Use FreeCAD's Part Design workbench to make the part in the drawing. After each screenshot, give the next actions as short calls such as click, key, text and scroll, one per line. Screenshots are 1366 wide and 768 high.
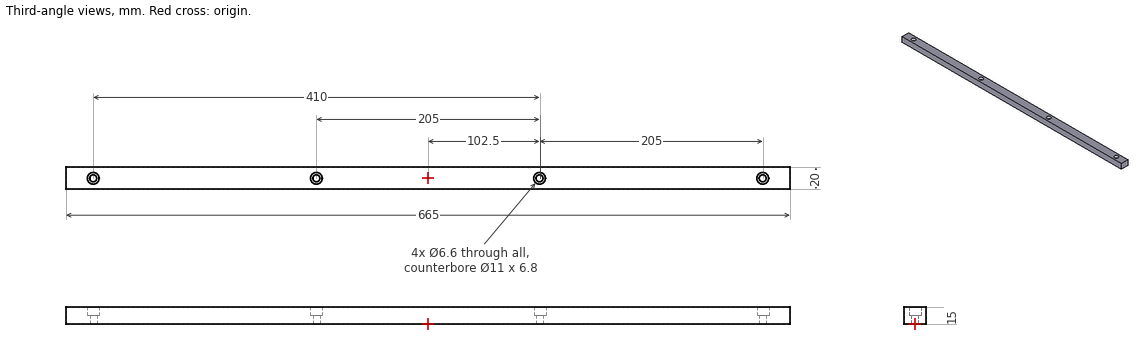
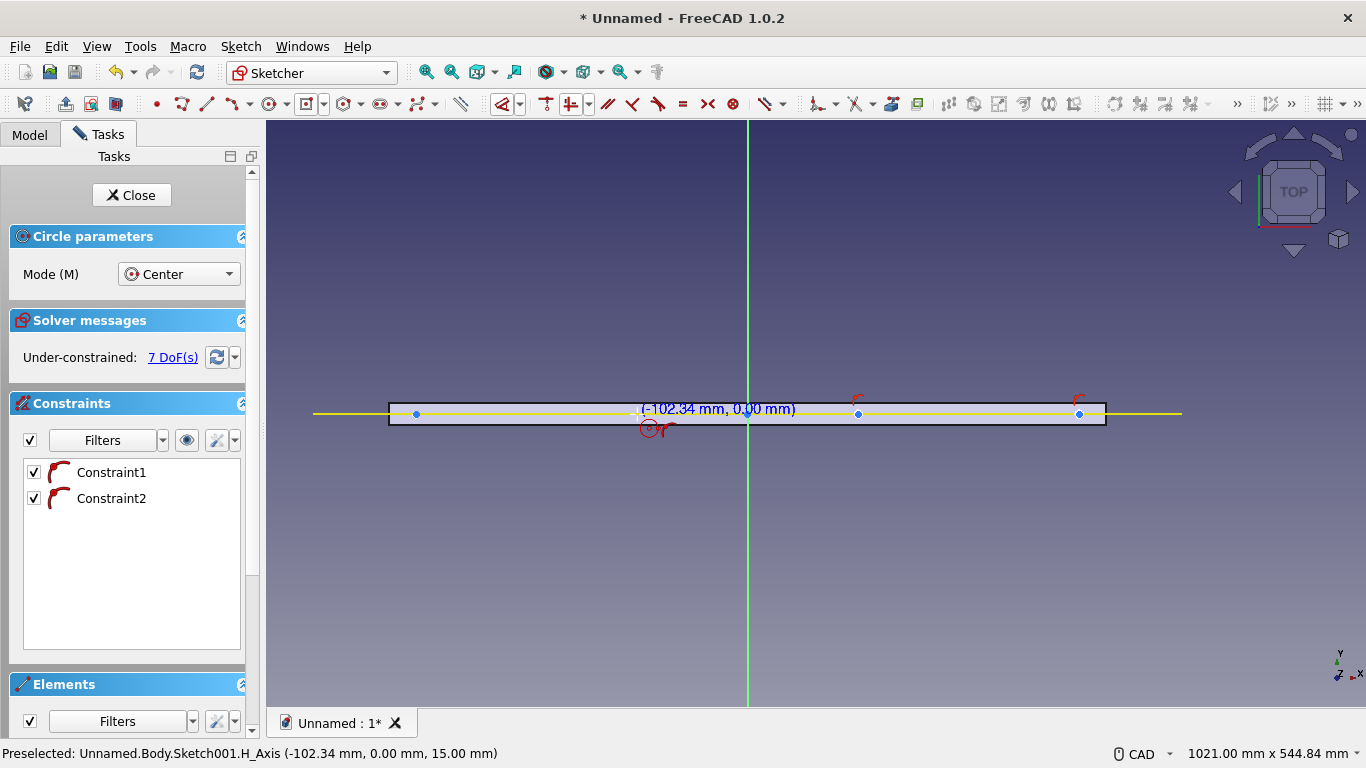
click(637, 414)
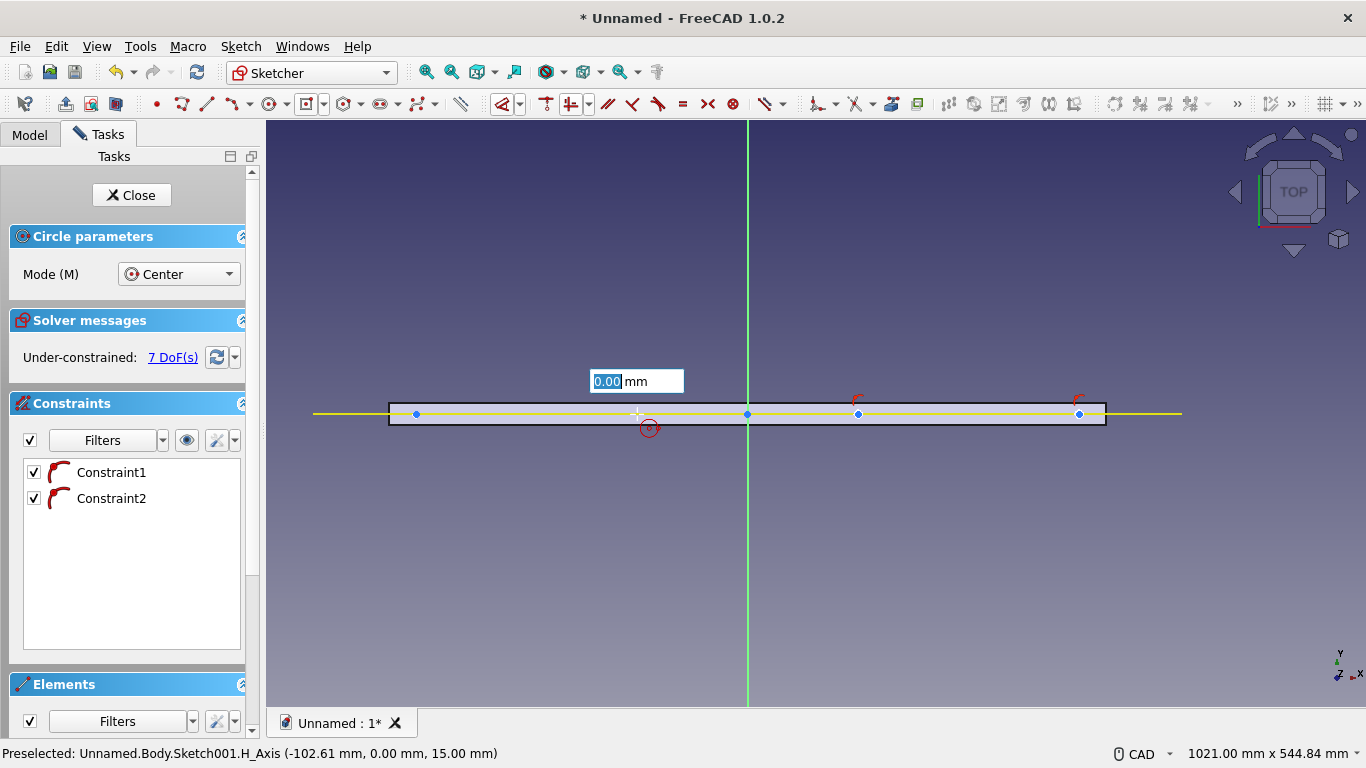
scroll(636, 417, up, 8)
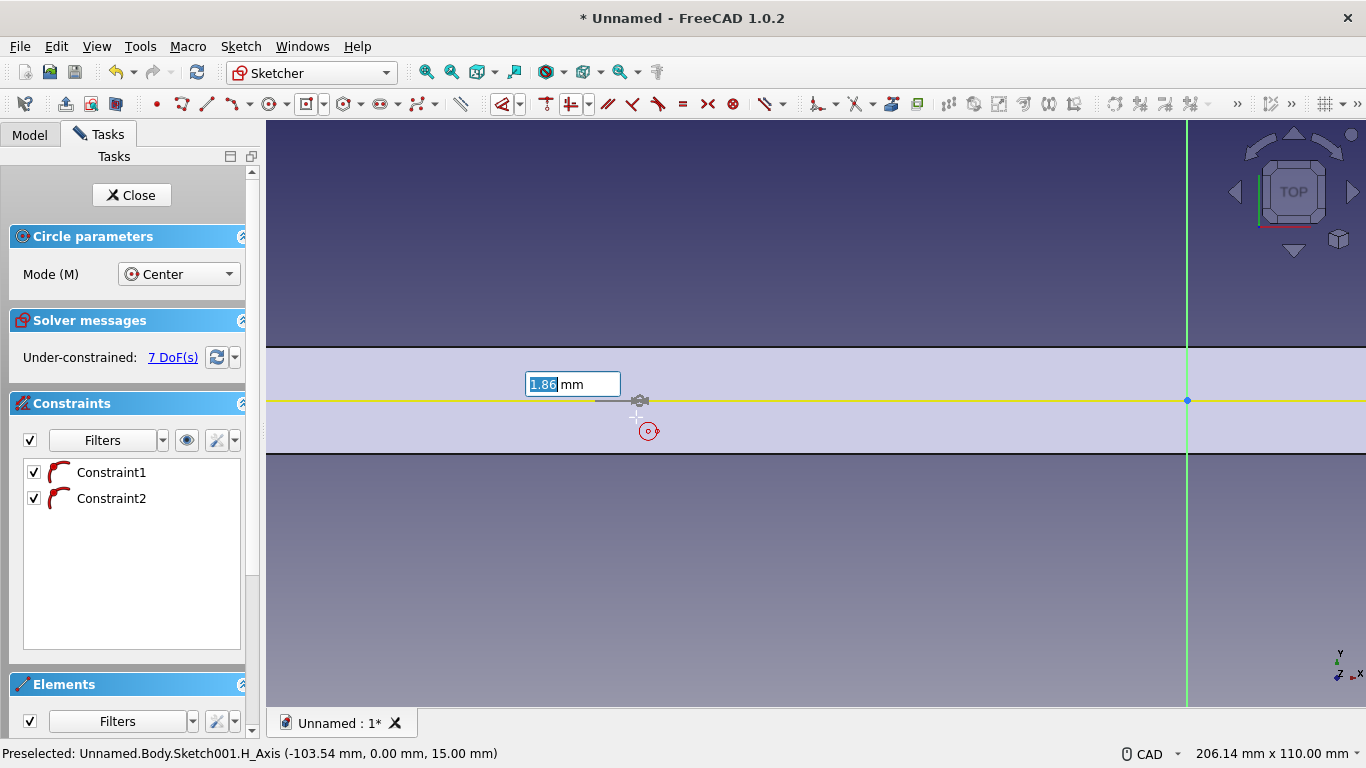
click(634, 417)
key(Escape)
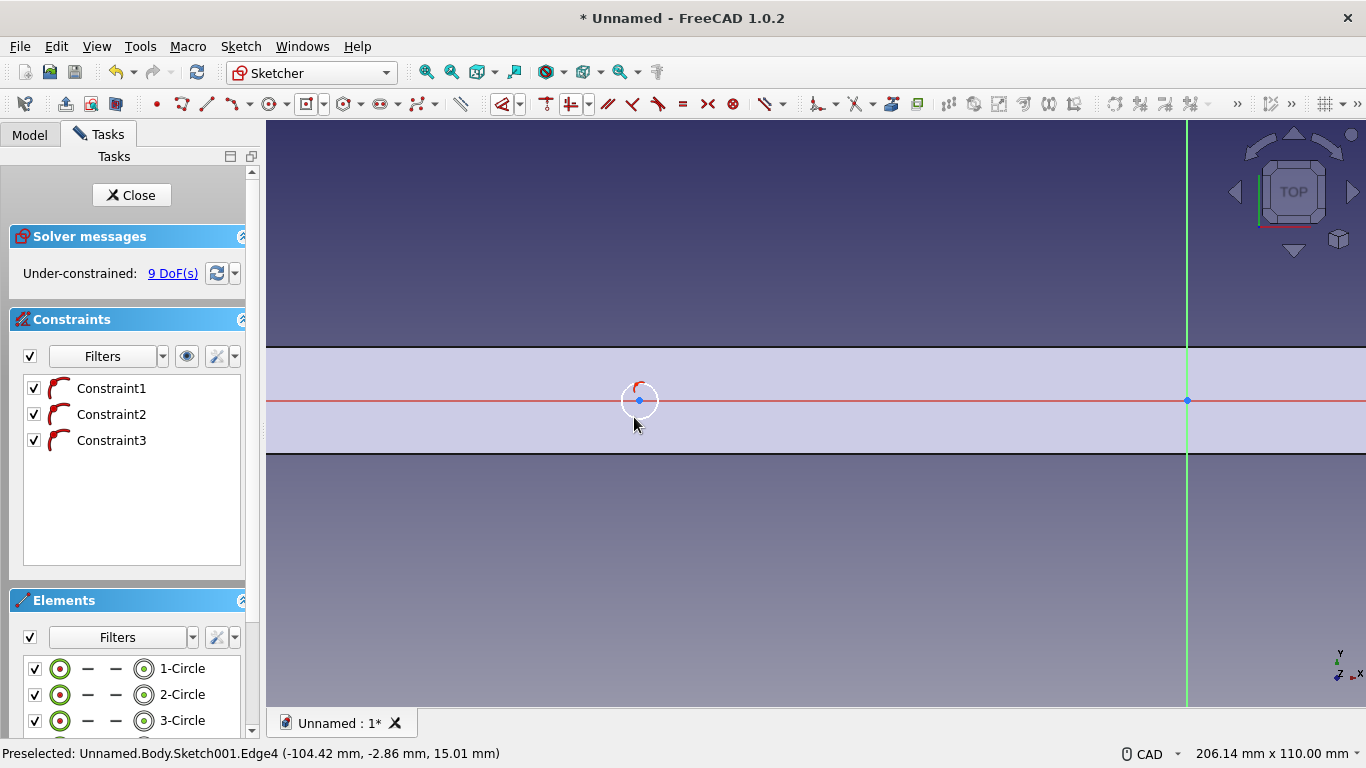
scroll(636, 417, down, 8)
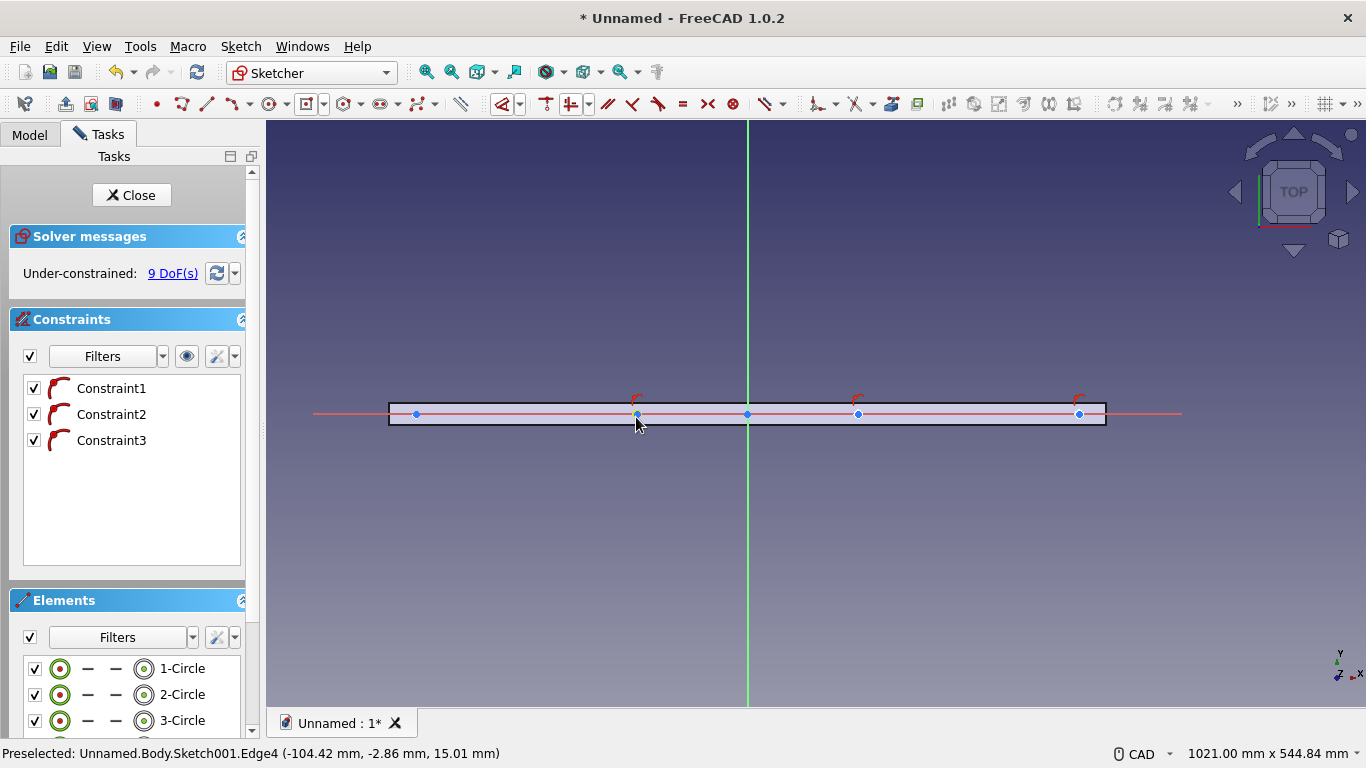
scroll(861, 412, up, 9)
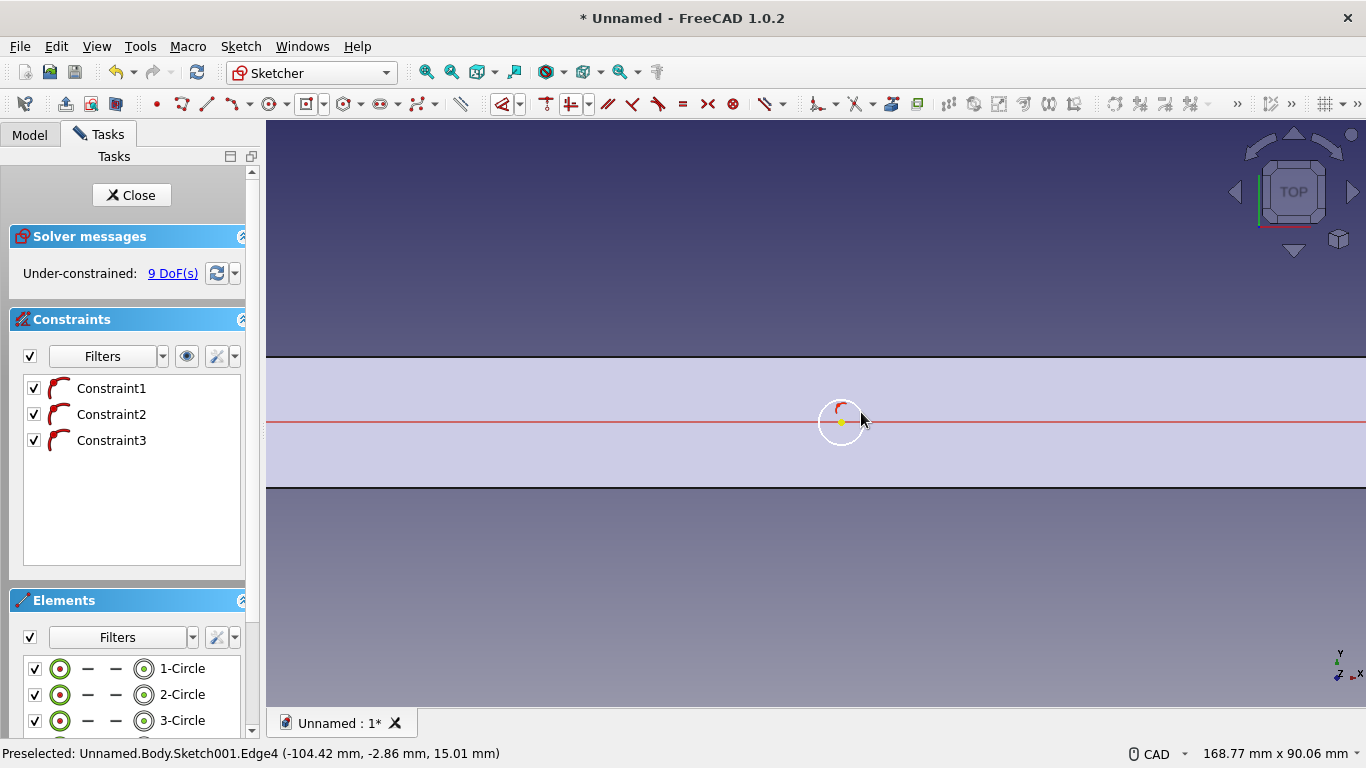
click(857, 406)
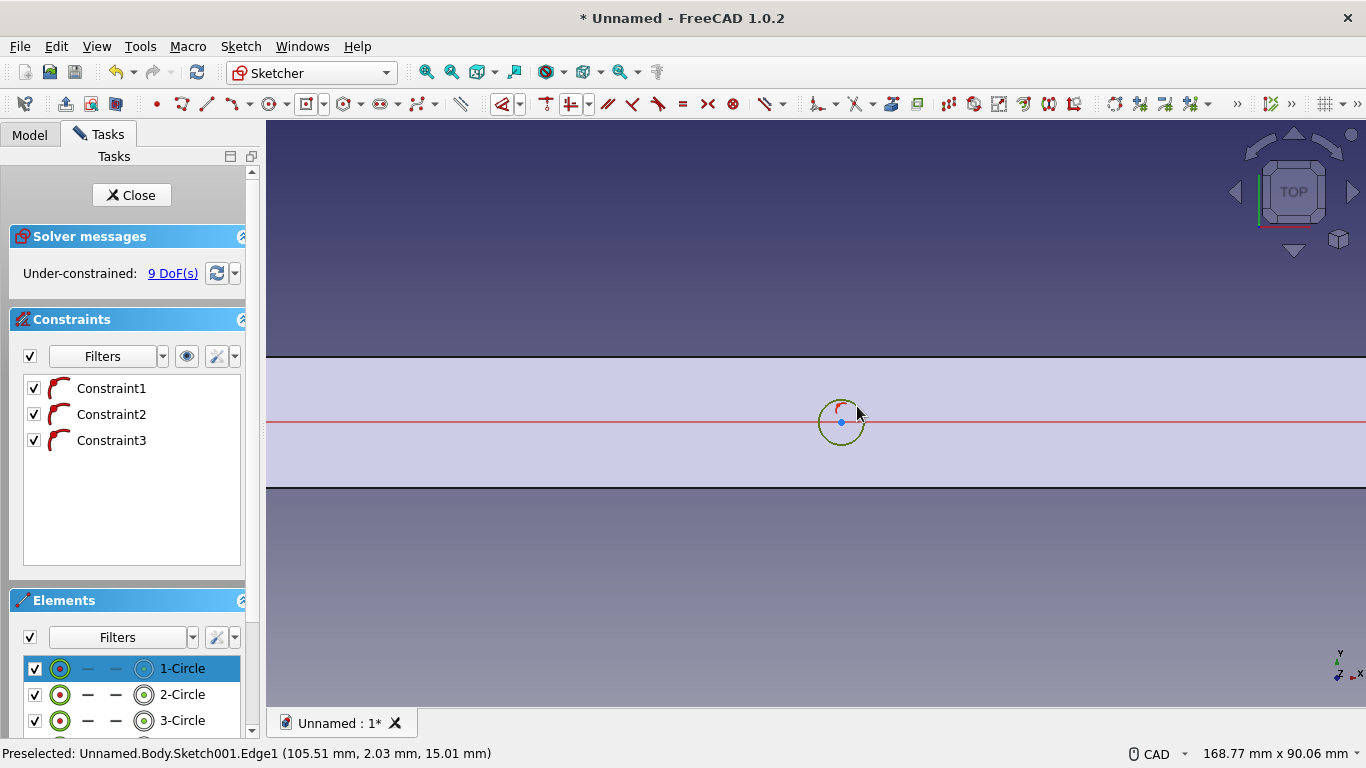
scroll(861, 412, down, 9)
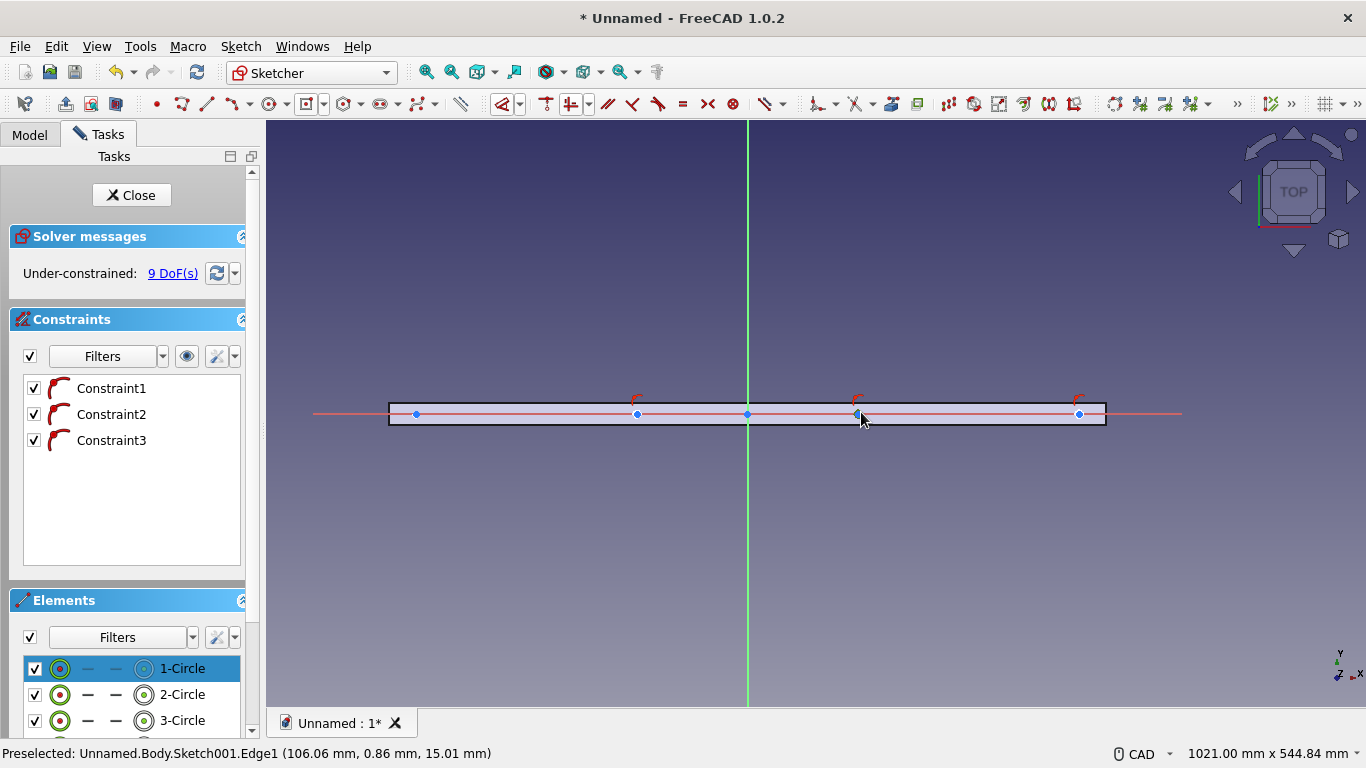
scroll(414, 417, up, 9)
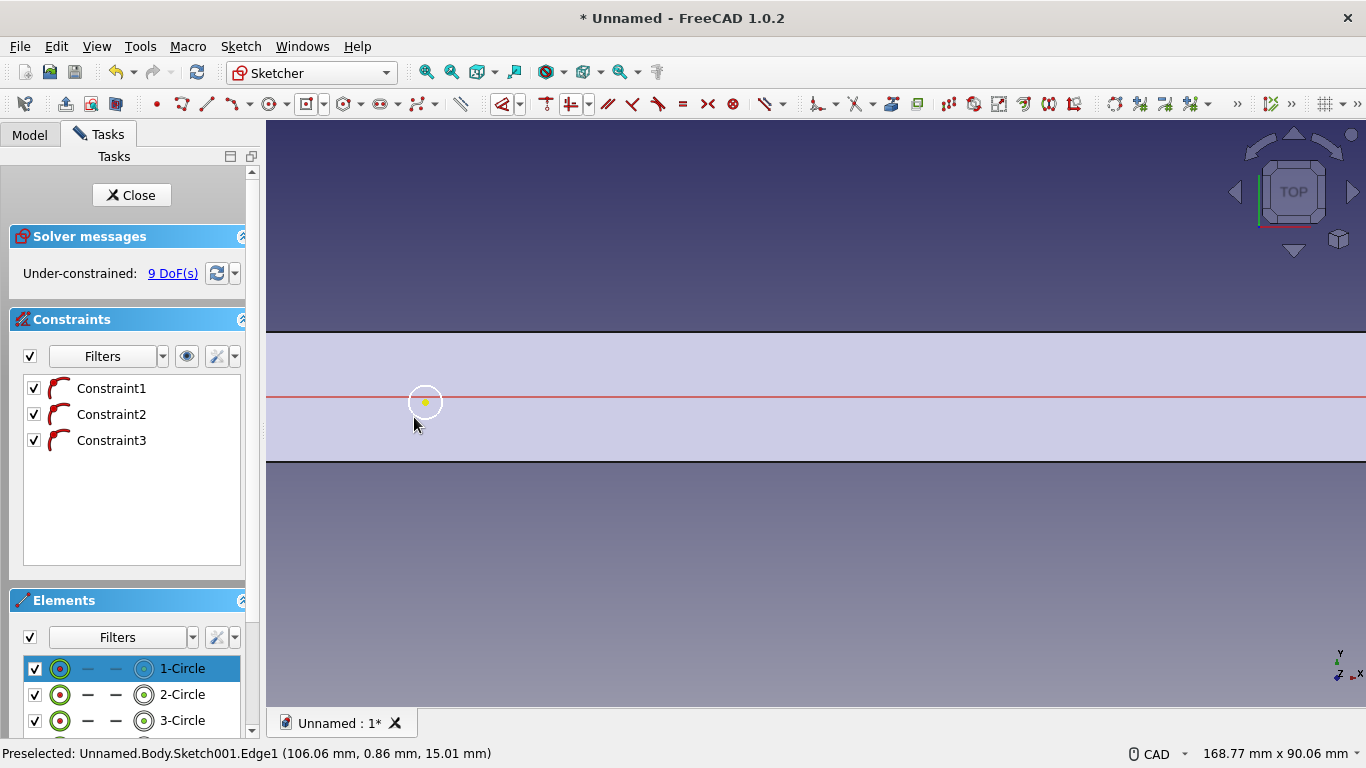
click(414, 414)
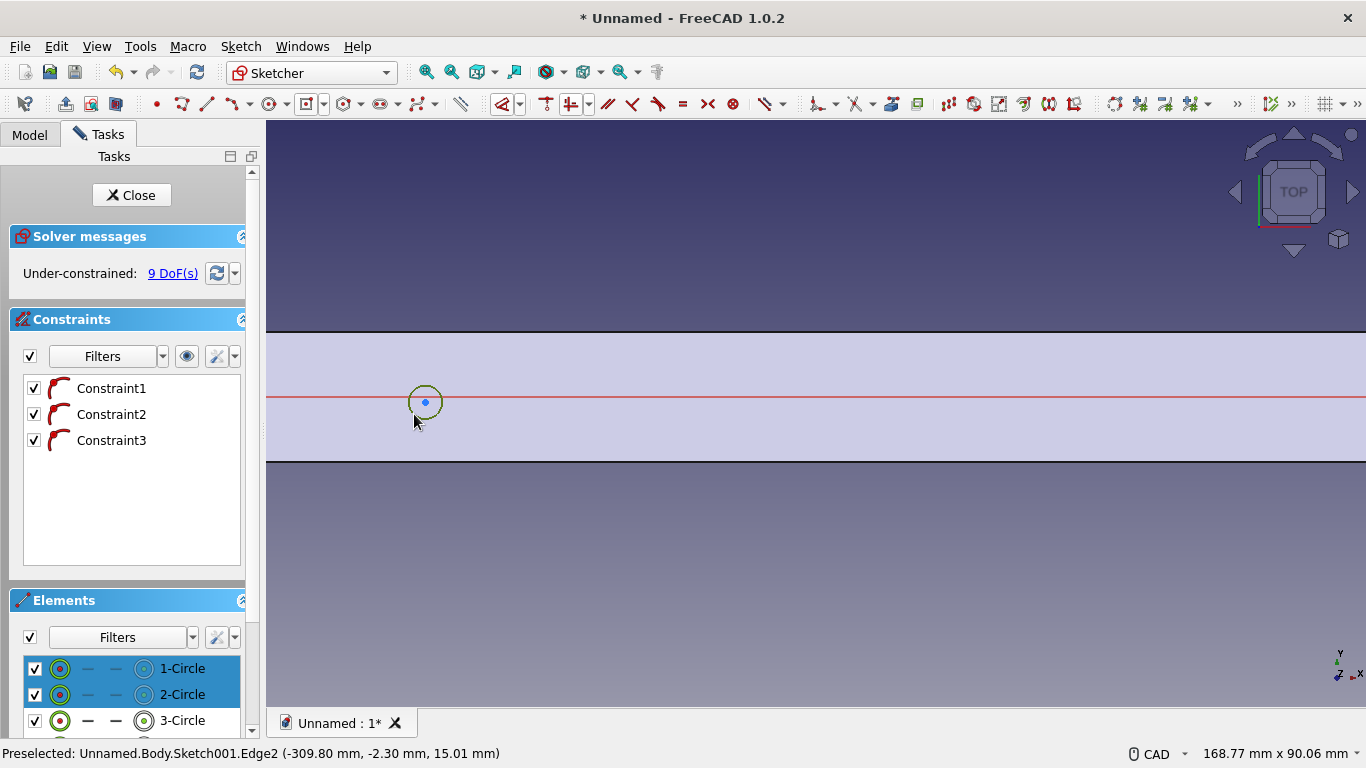
scroll(414, 417, down, 9)